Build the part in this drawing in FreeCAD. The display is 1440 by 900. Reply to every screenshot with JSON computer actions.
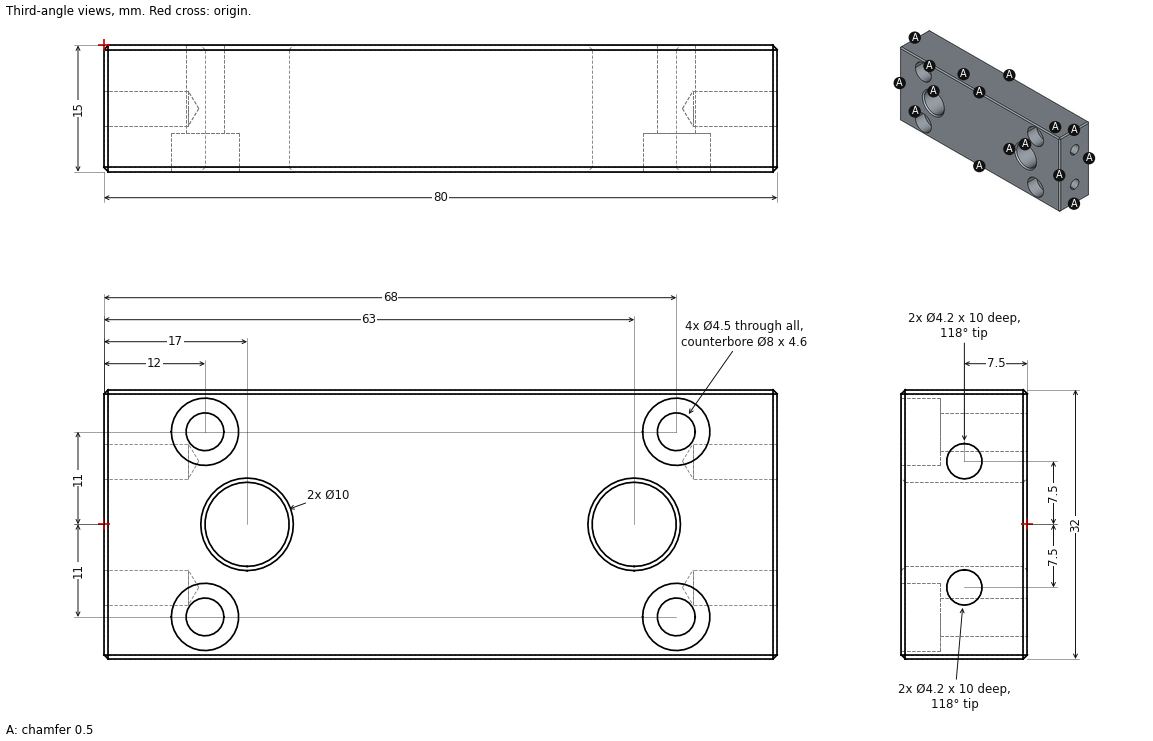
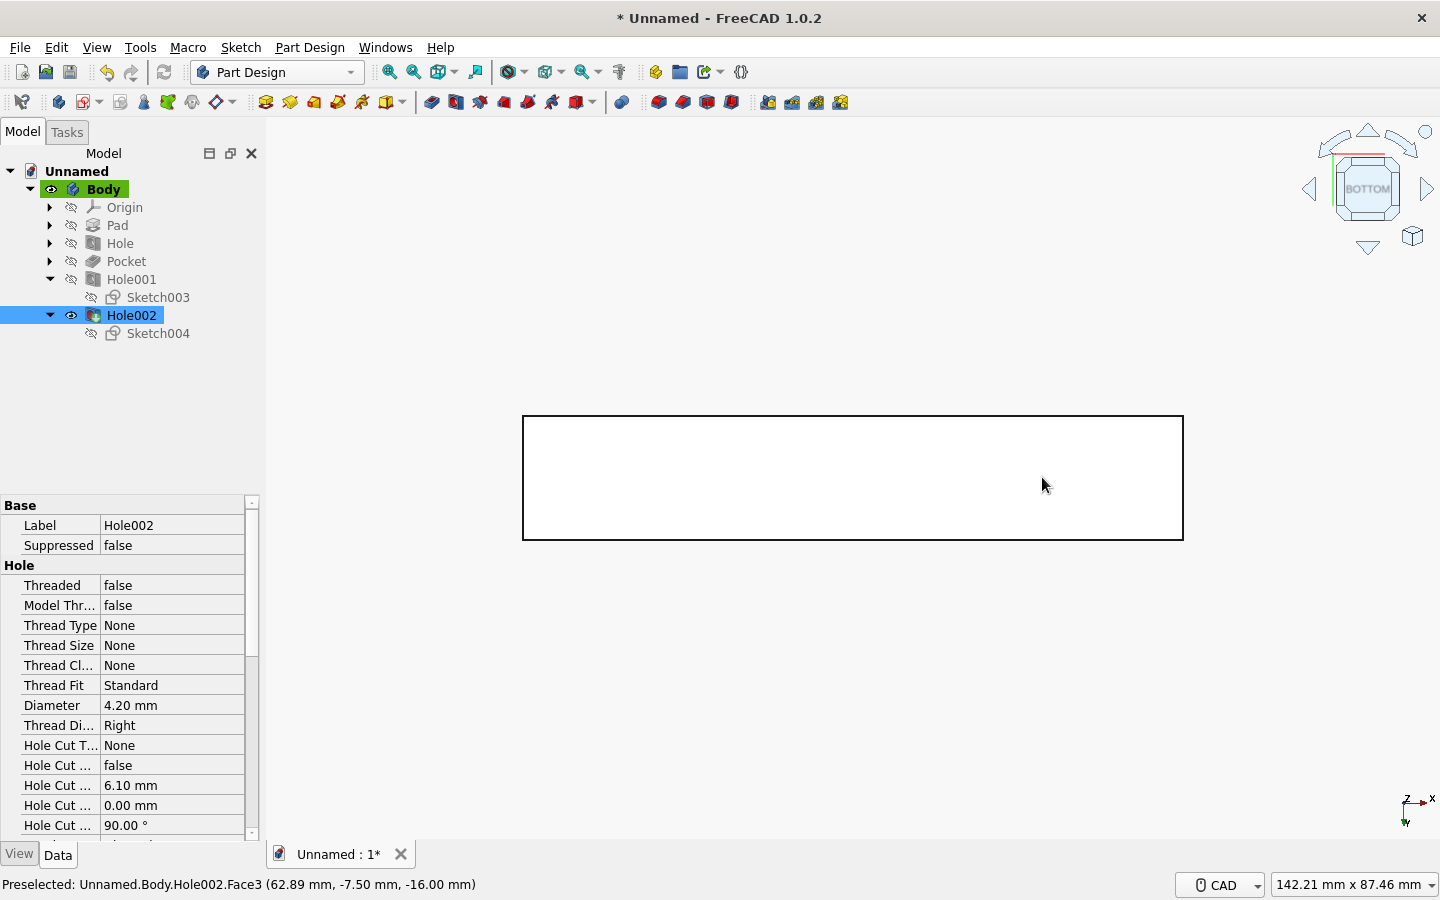
{"action": "key", "text": "4"}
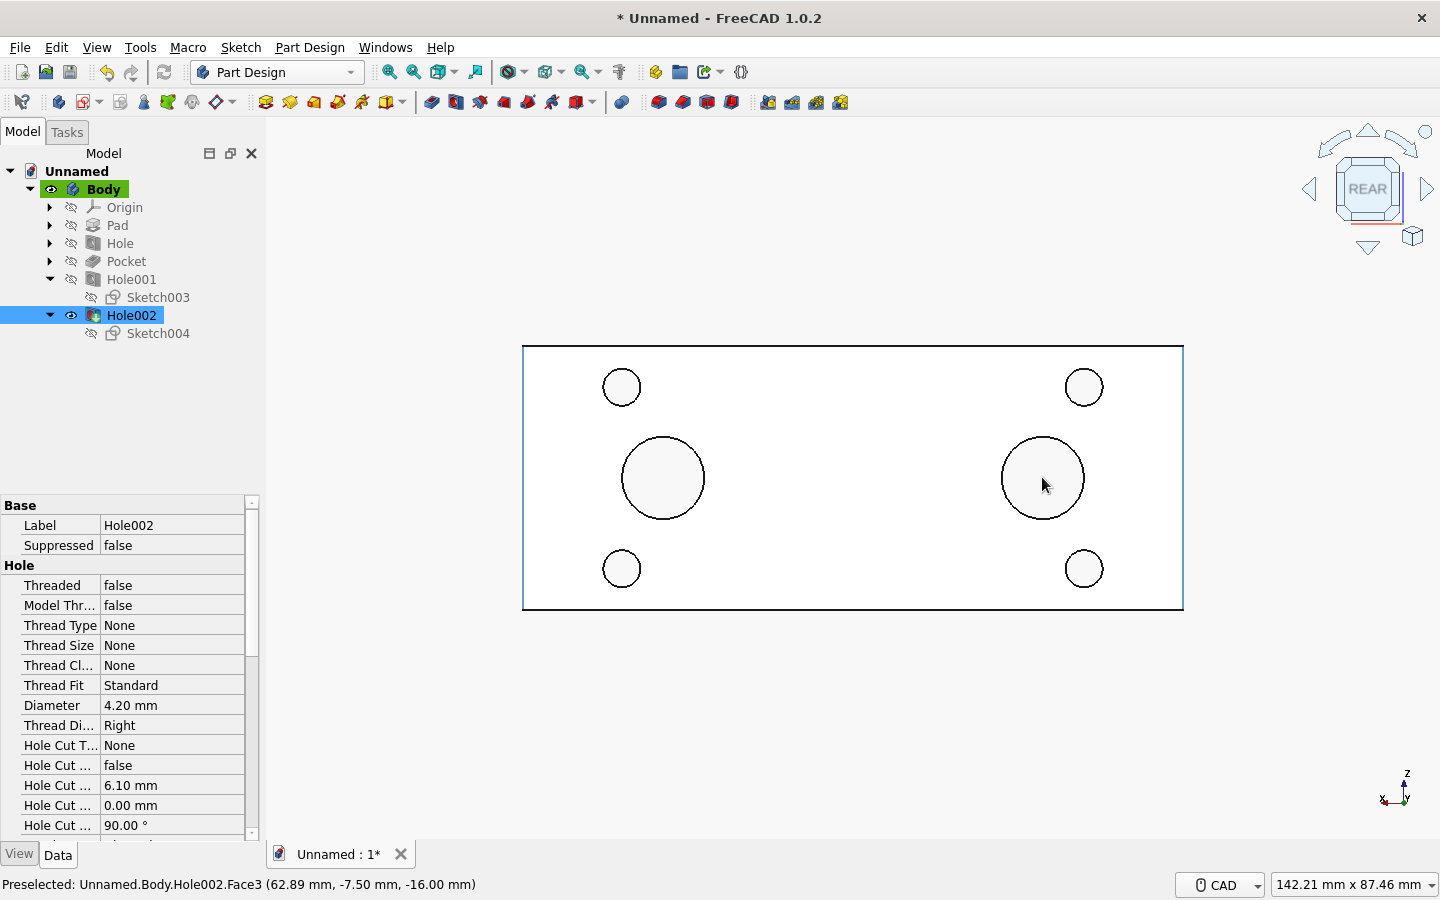
{"action": "left_click", "coordinate": [1084, 477], "text": "ctrl"}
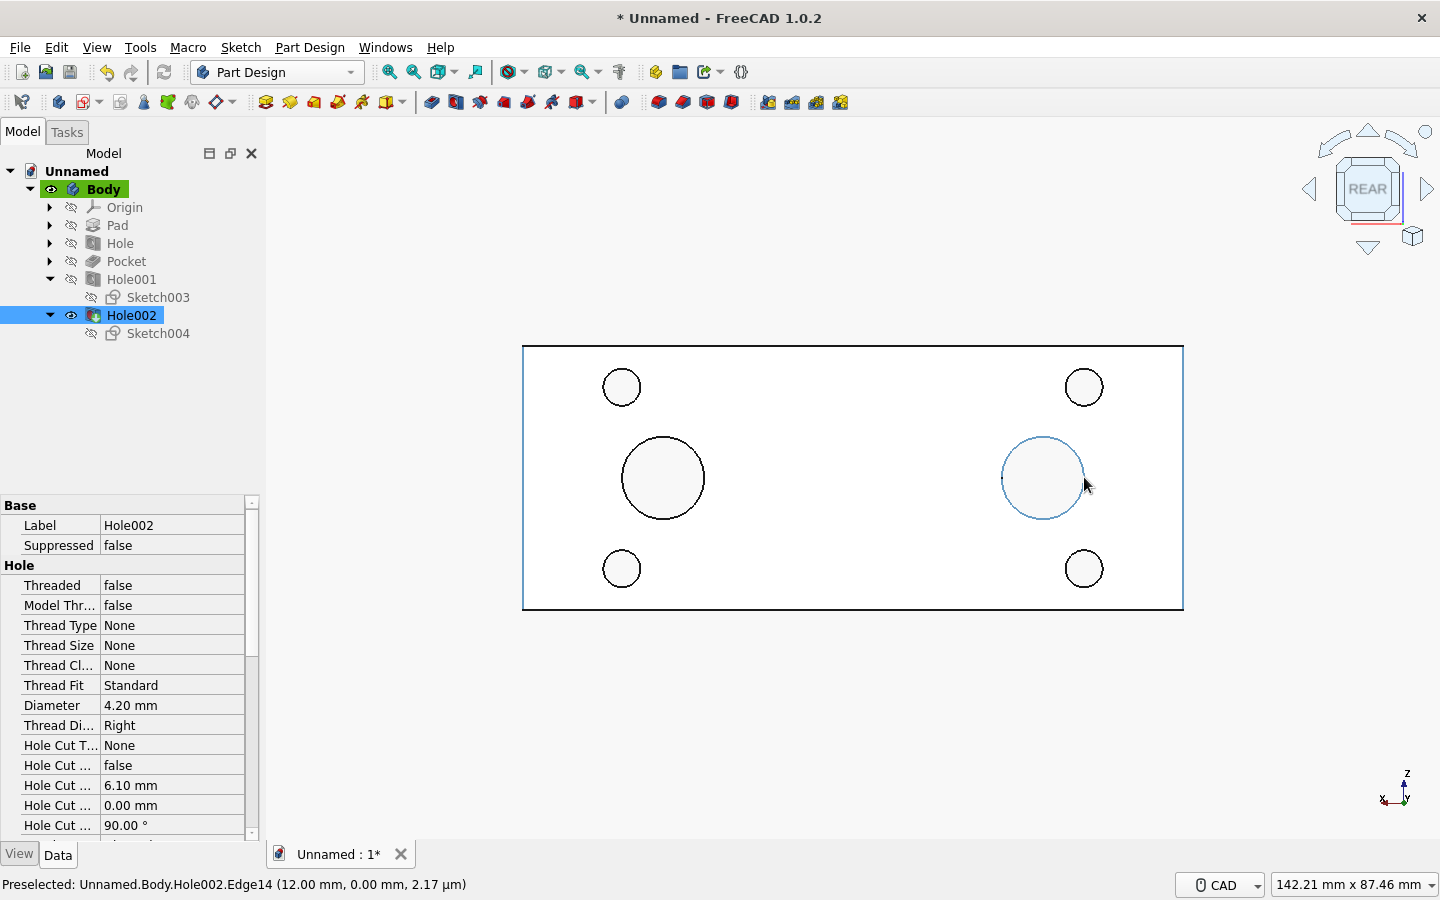
{"action": "left_click", "coordinate": [704, 477], "text": "ctrl"}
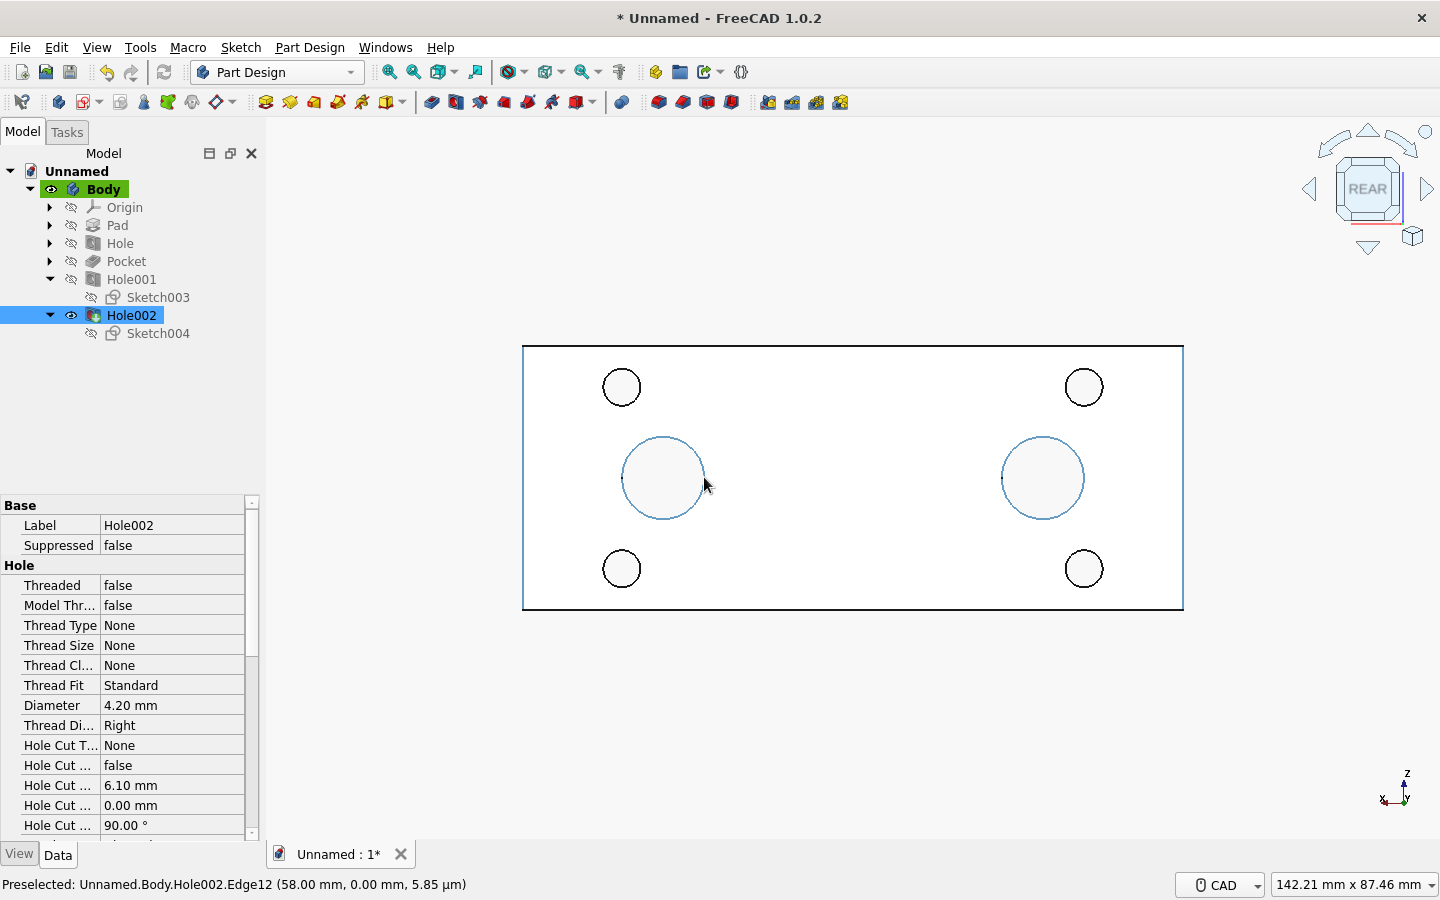
{"action": "left_click", "coordinate": [684, 102]}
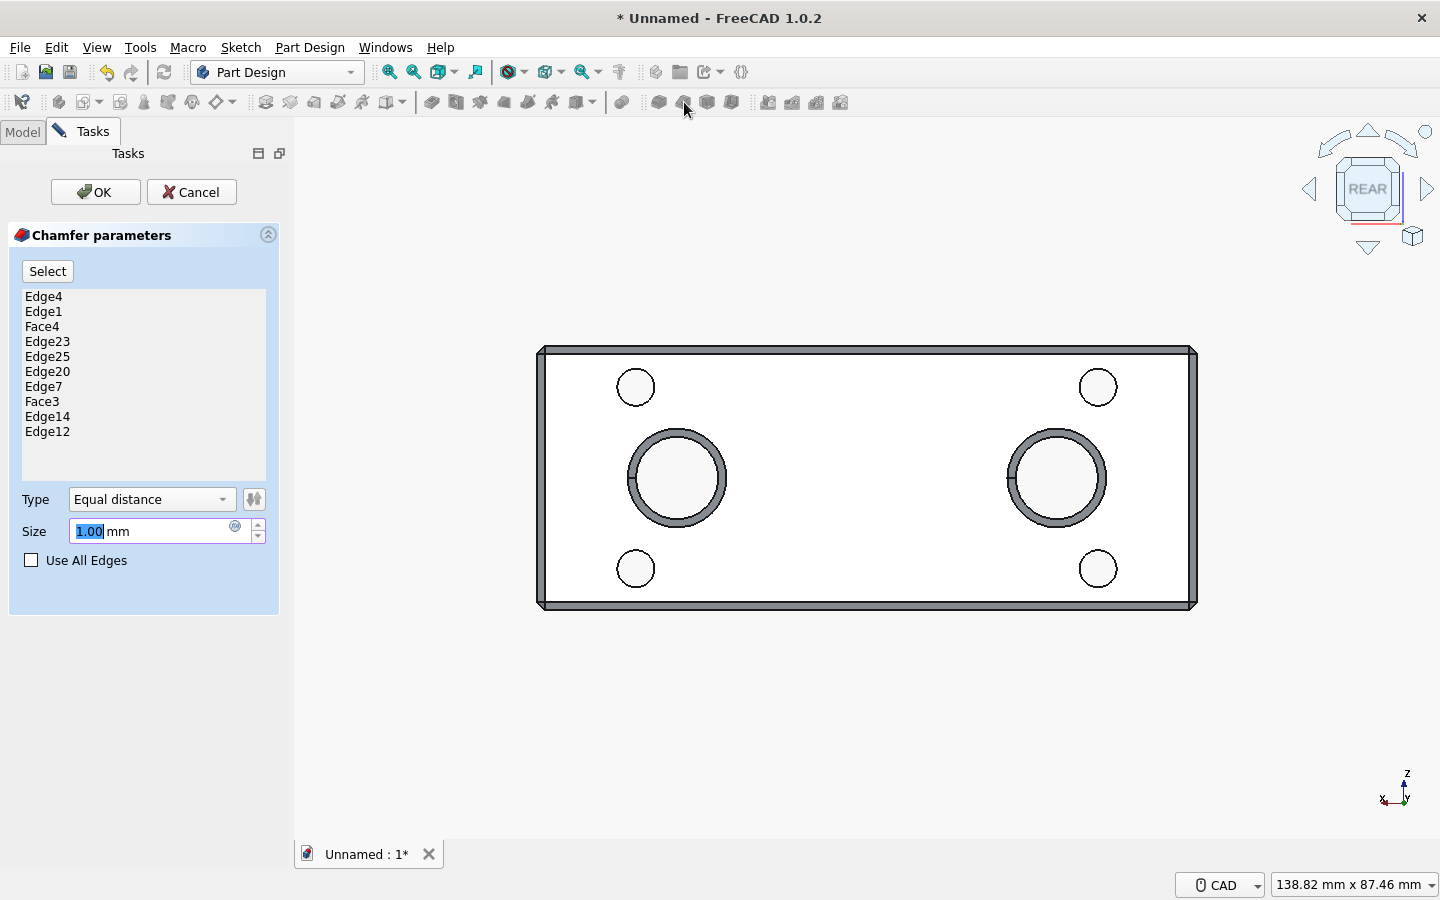
{"action": "type", "text": "0.5"}
{"action": "key", "text": "Tab"}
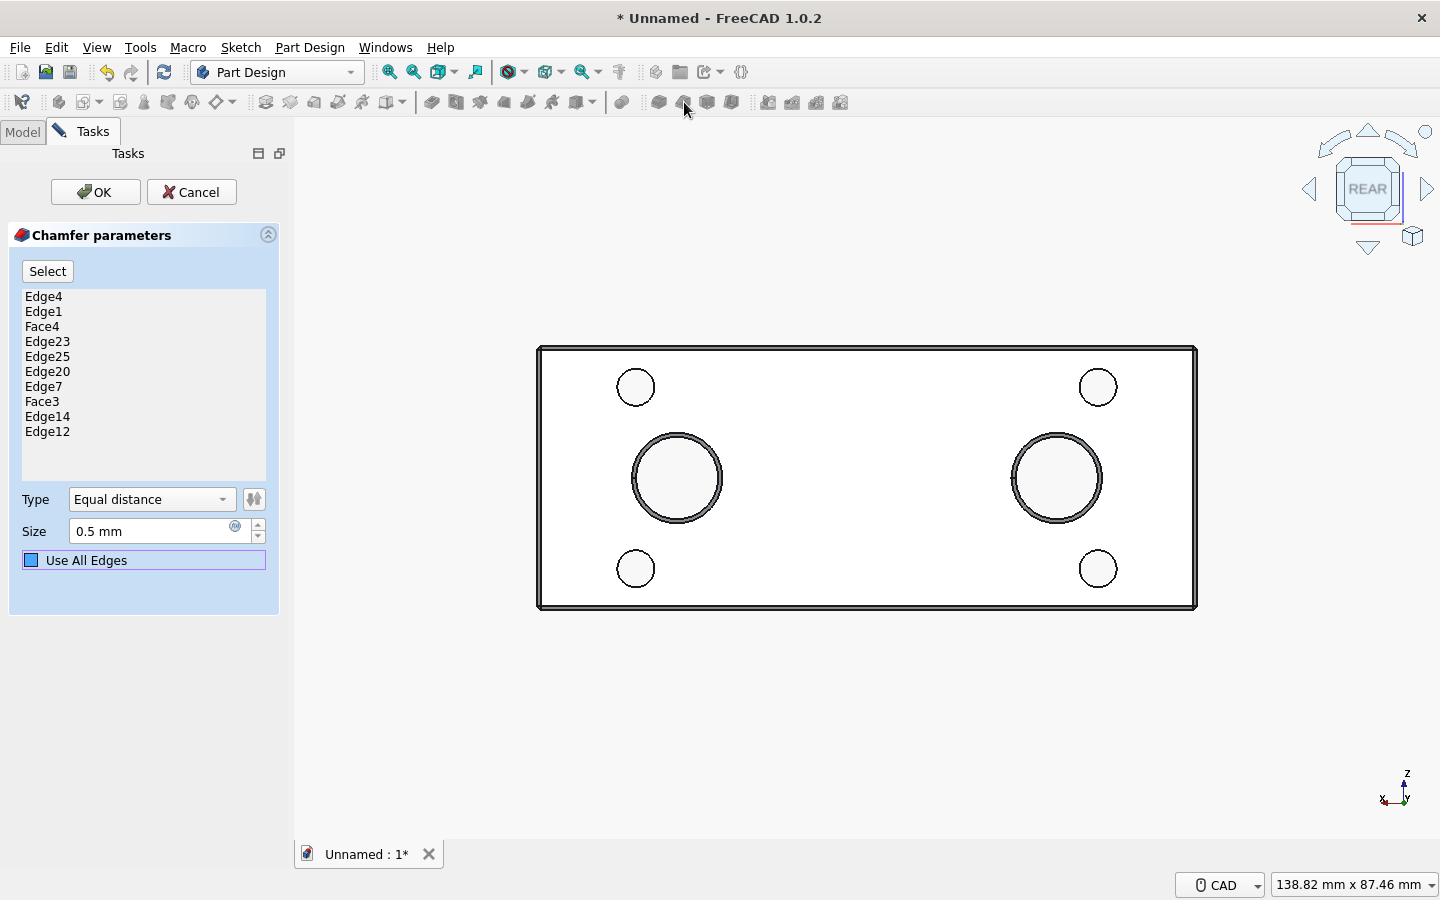
{"action": "left_click", "coordinate": [96, 192]}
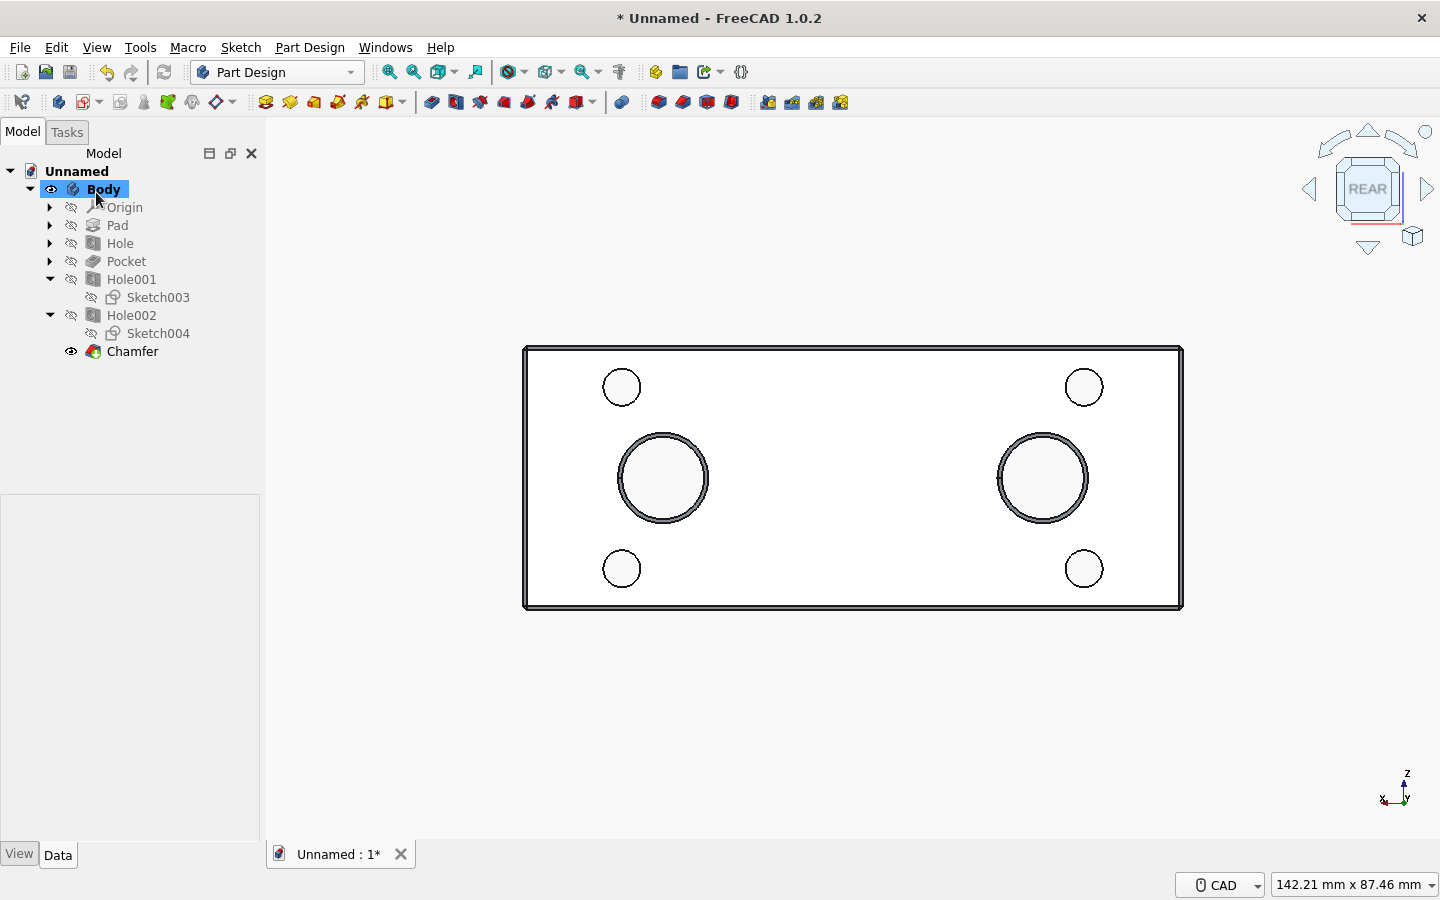
{"action": "key", "text": "0"}